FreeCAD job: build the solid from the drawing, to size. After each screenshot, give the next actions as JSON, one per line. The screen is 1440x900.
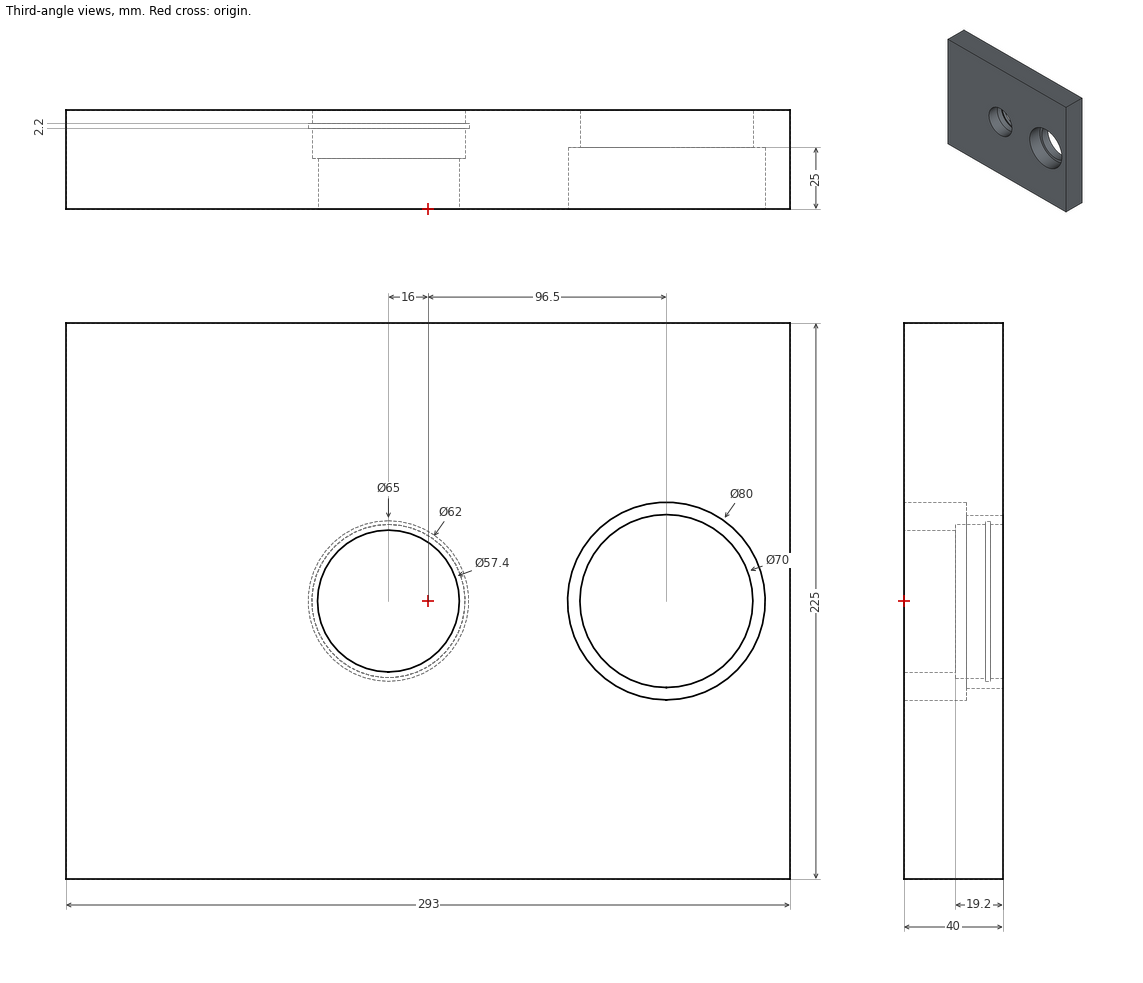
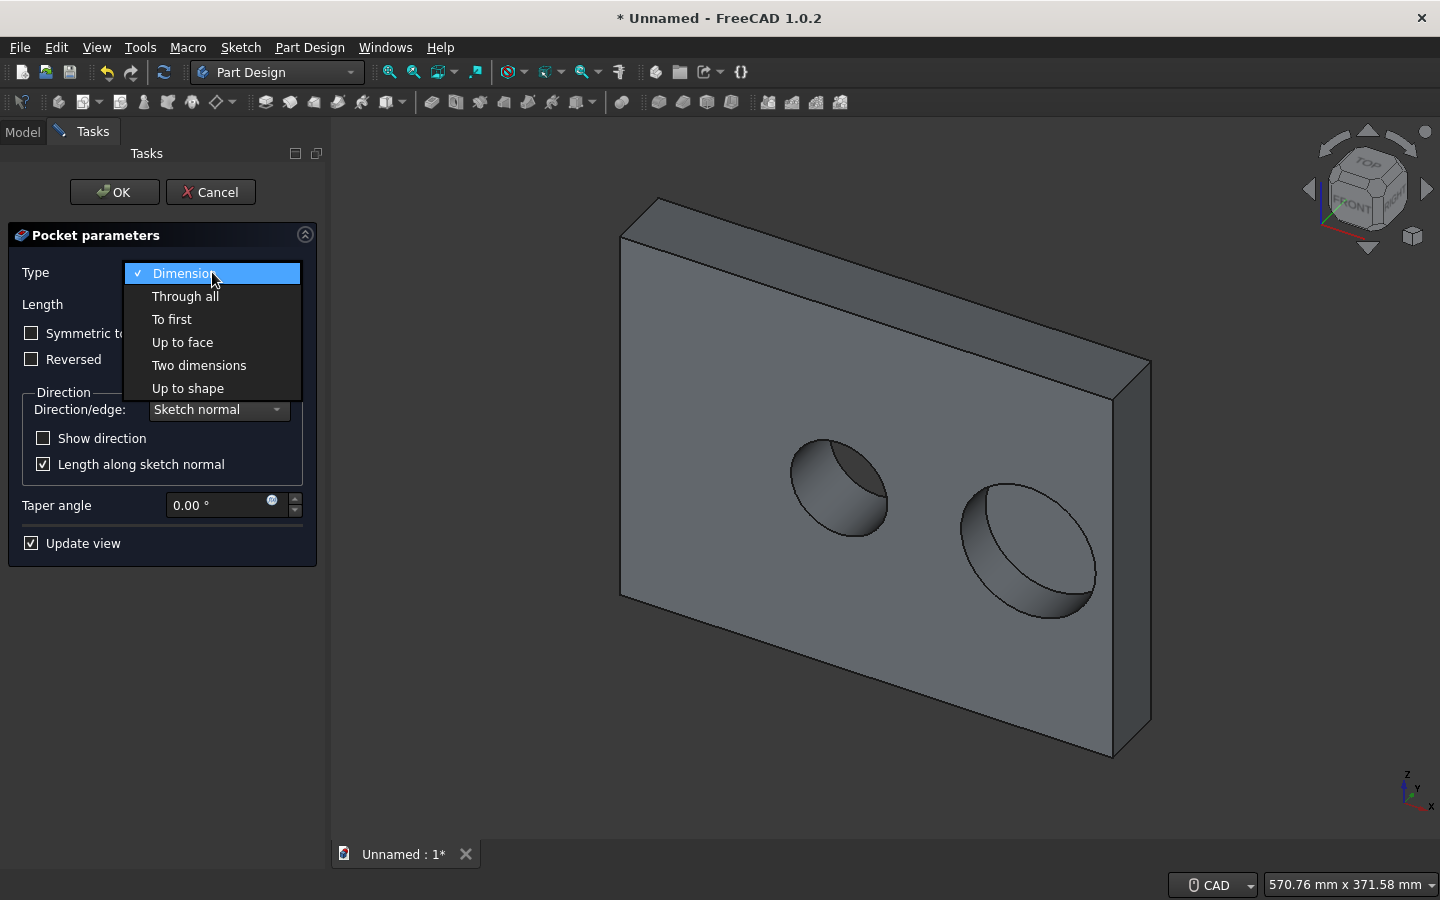
{"action": "left_click", "coordinate": [212, 296]}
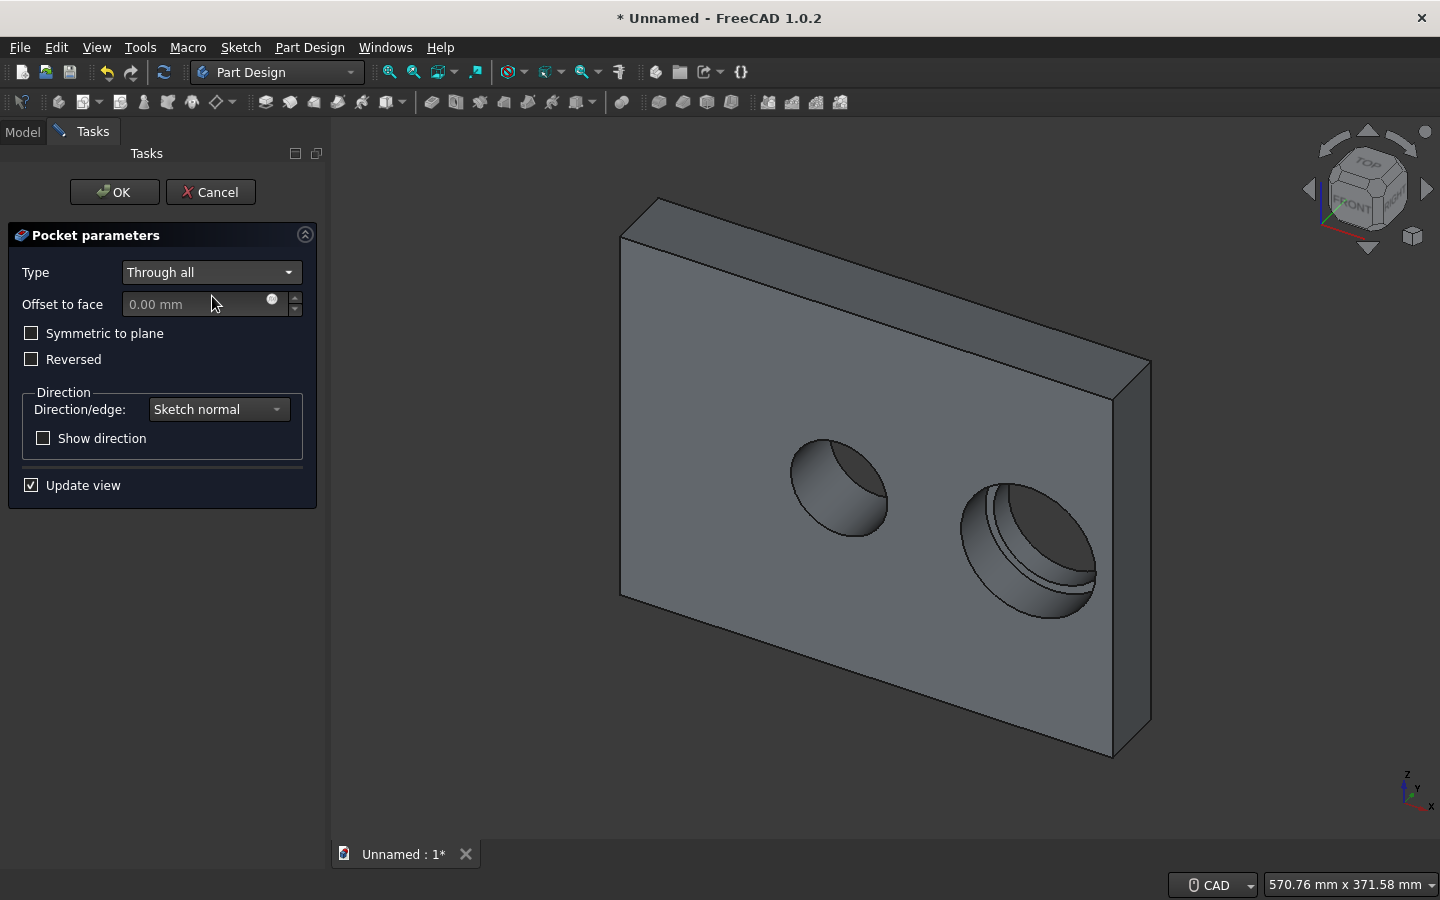
{"action": "left_click", "coordinate": [115, 192]}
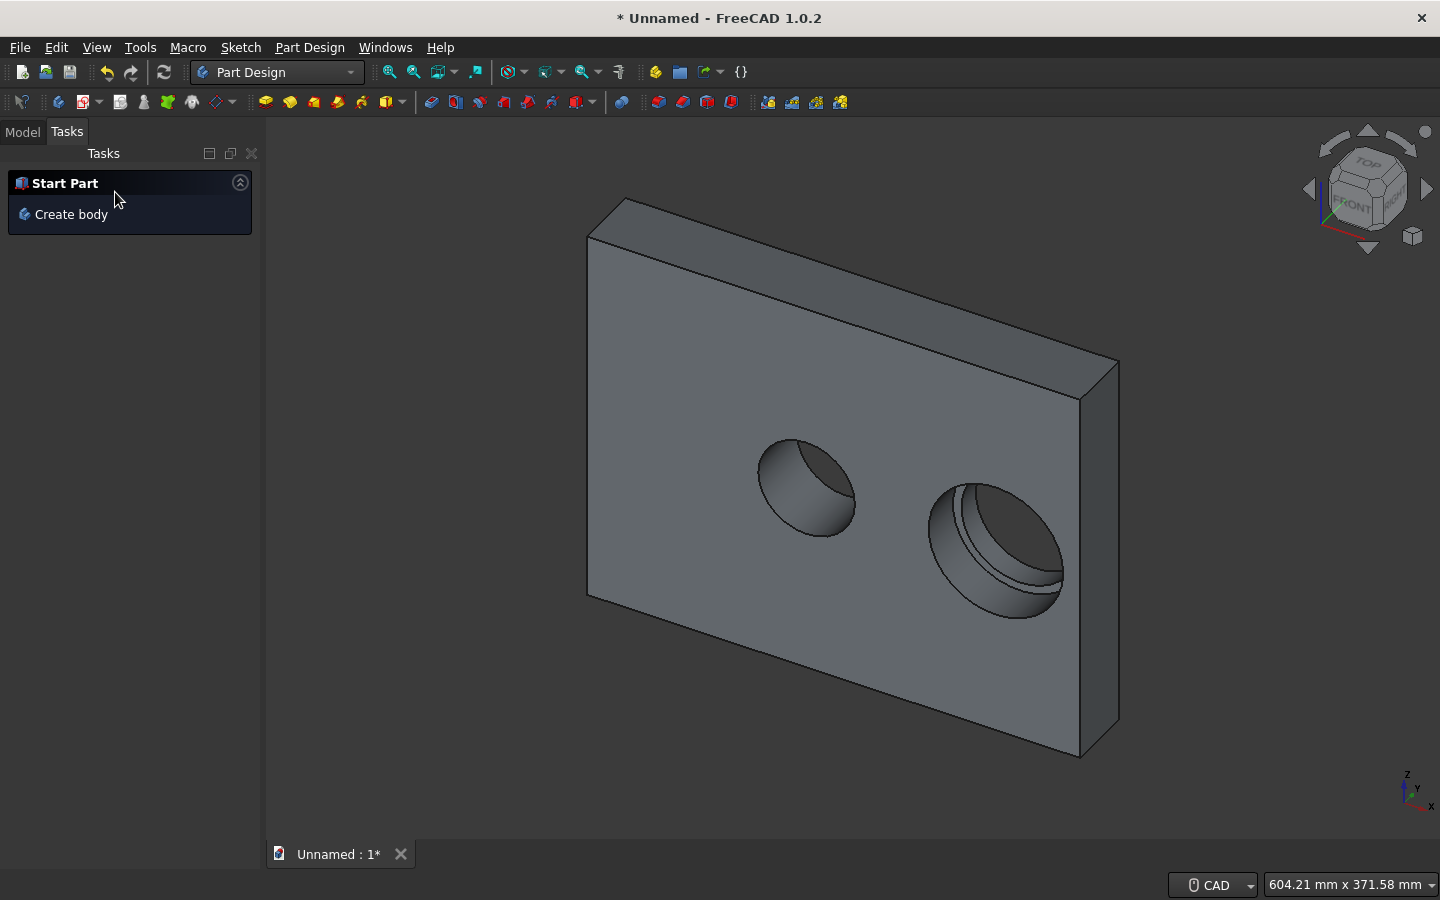
{"action": "key", "text": "4"}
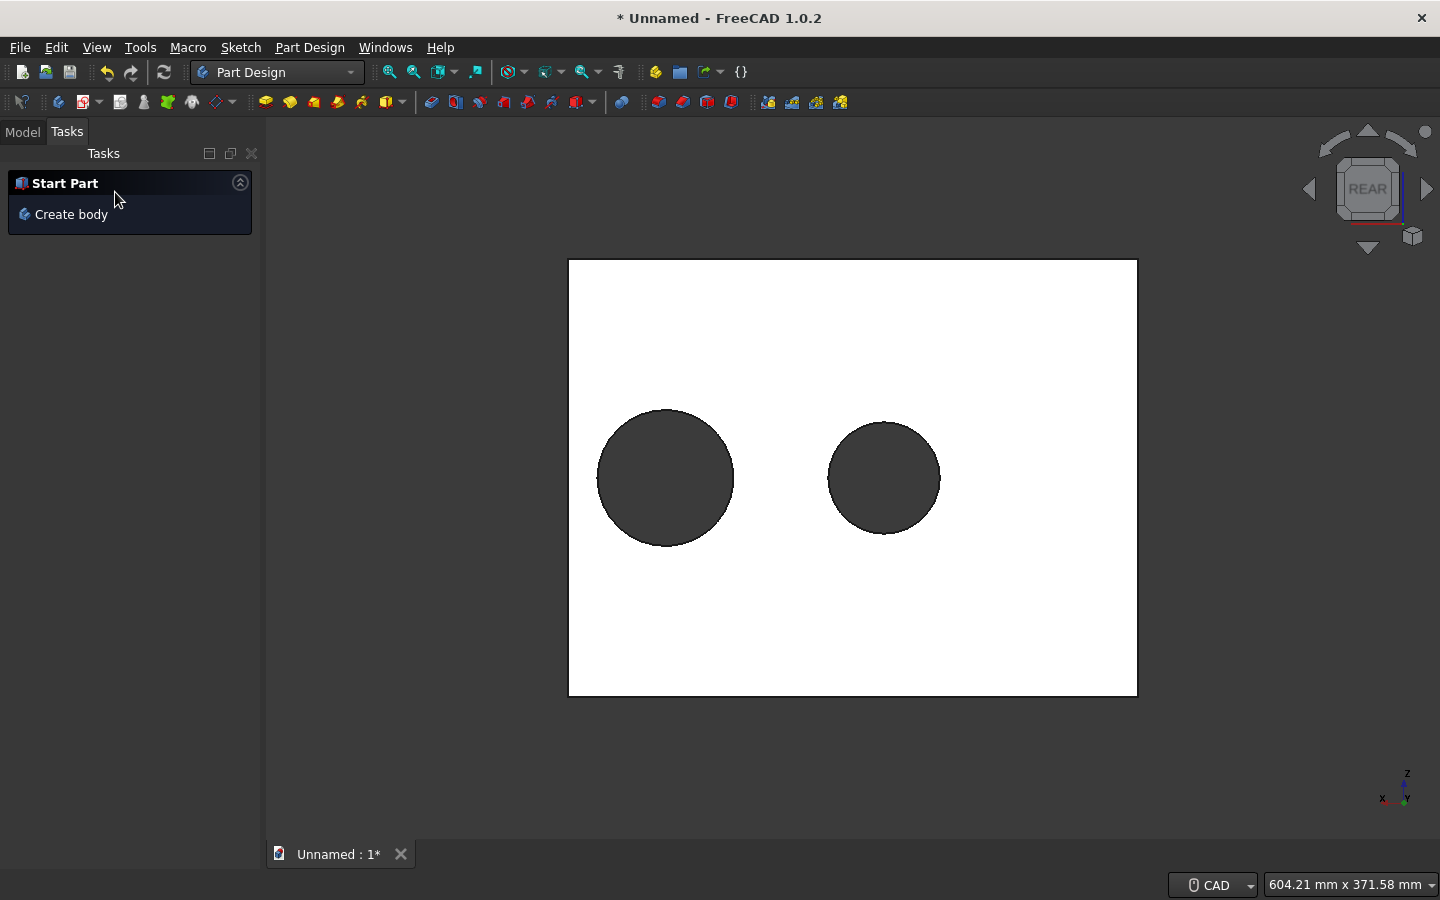
{"action": "left_click", "coordinate": [772, 352]}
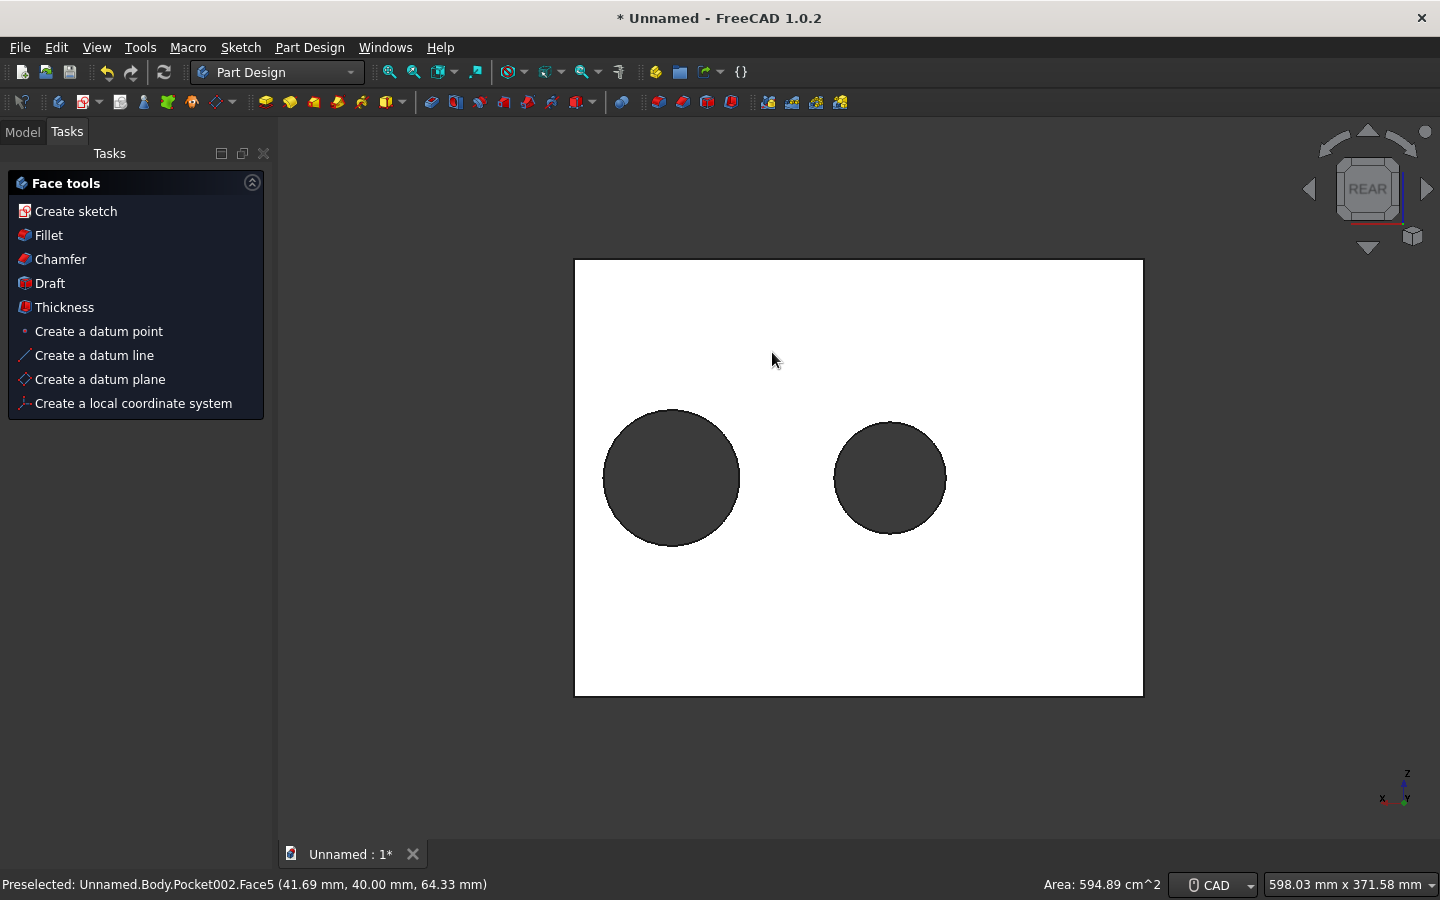
{"action": "left_click", "coordinate": [84, 102]}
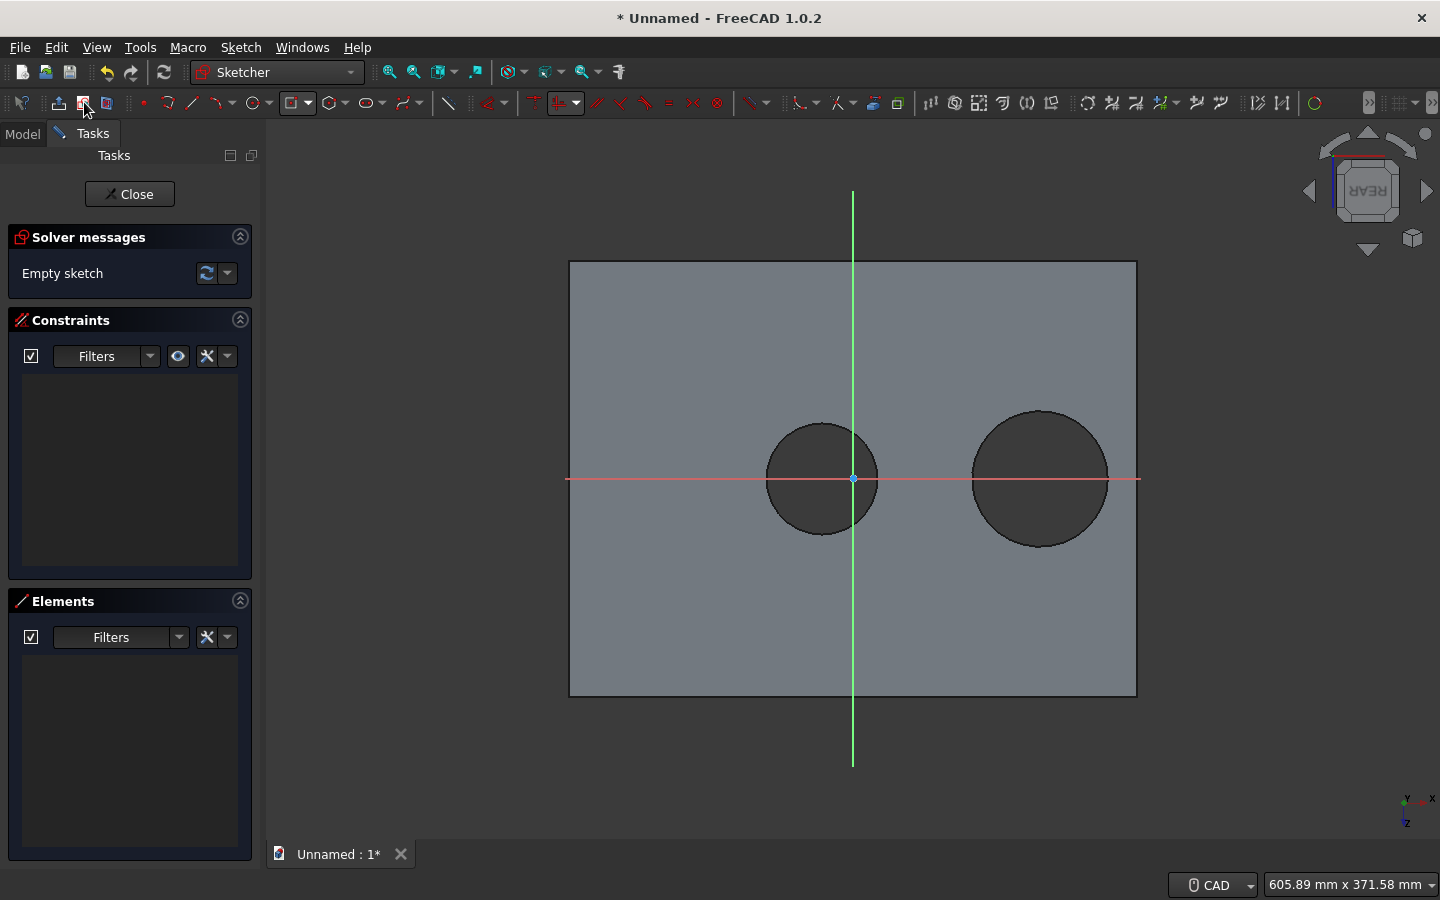
{"action": "scroll", "coordinate": [834, 479], "scroll_direction": "up", "scroll_amount": 7}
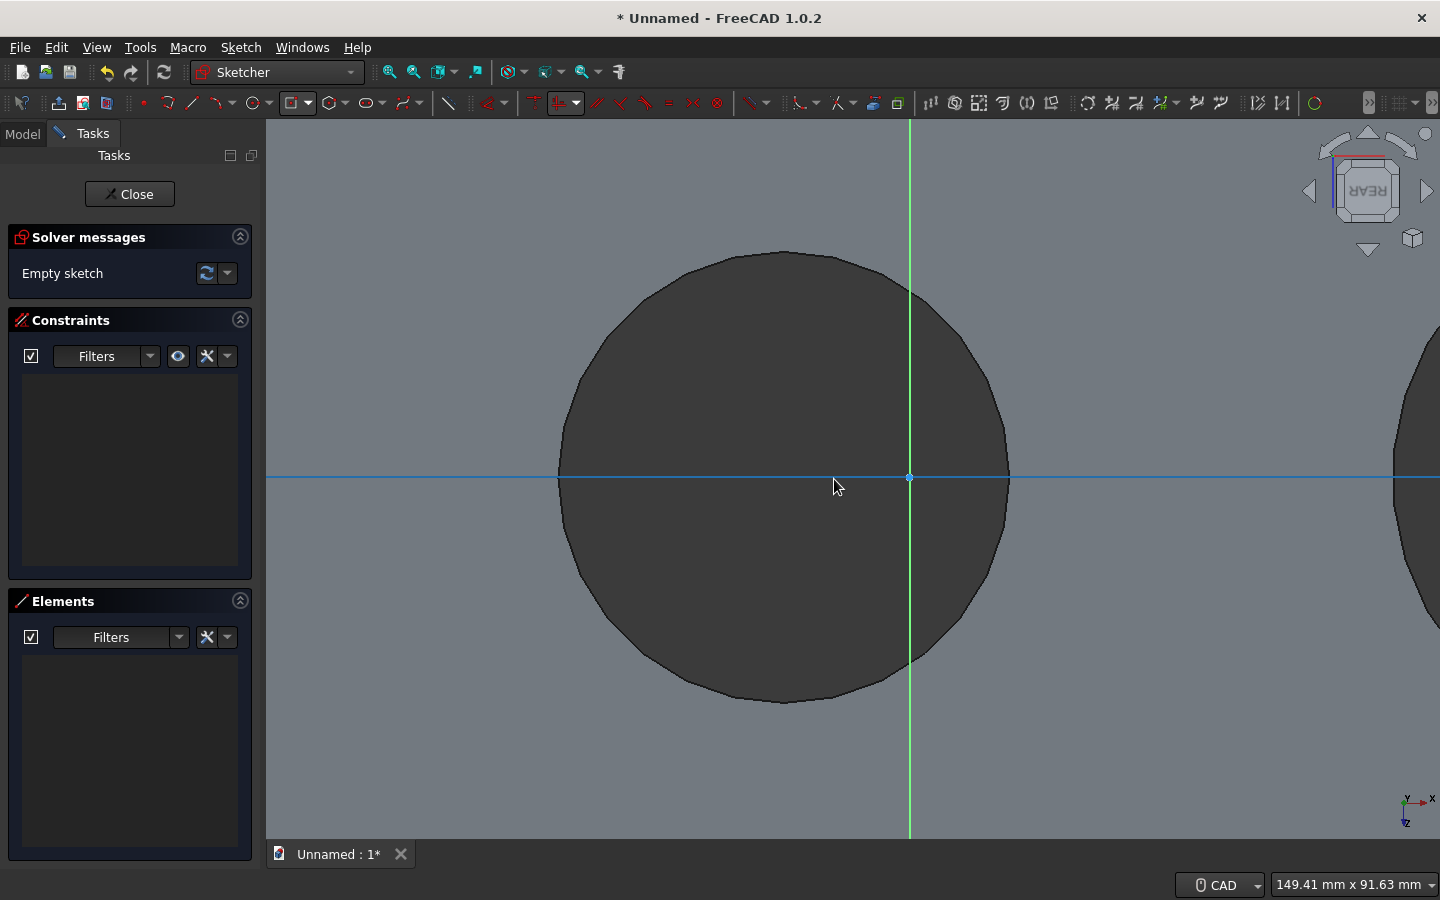
{"action": "left_click", "coordinate": [254, 104]}